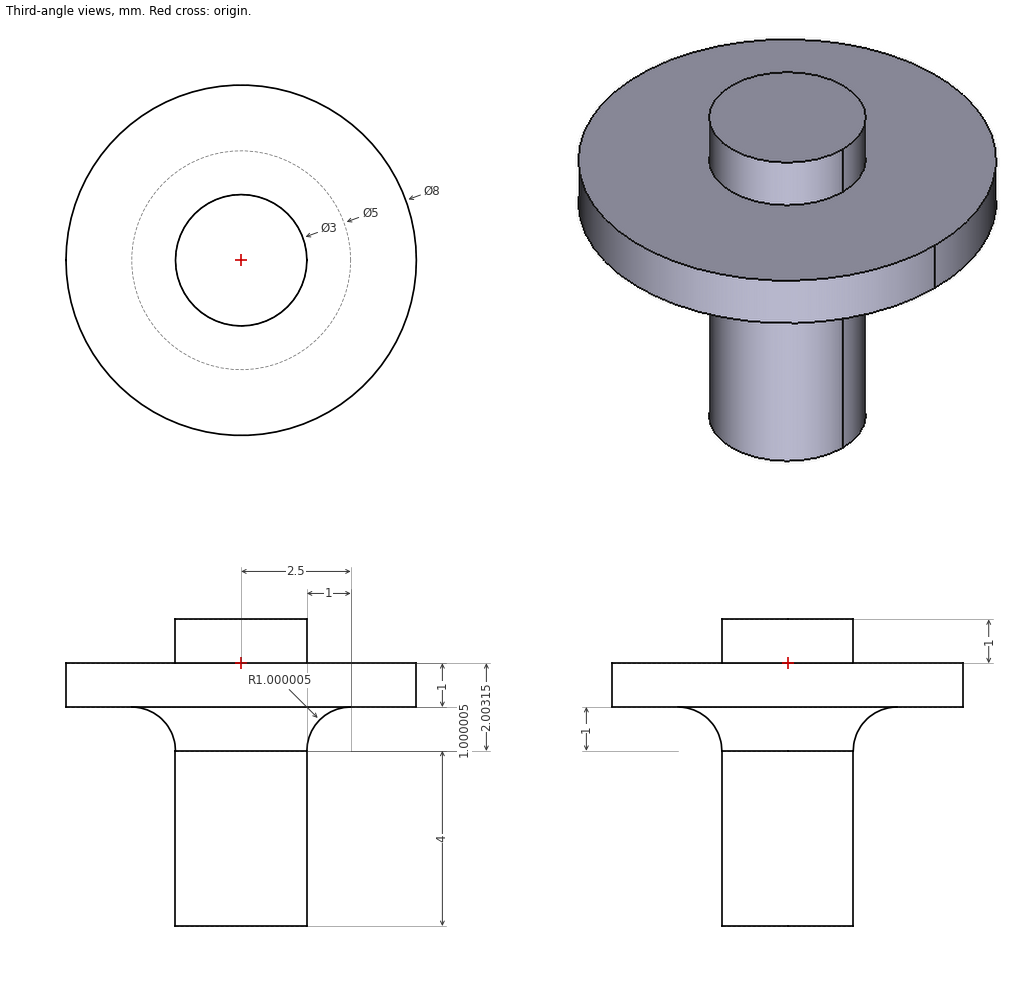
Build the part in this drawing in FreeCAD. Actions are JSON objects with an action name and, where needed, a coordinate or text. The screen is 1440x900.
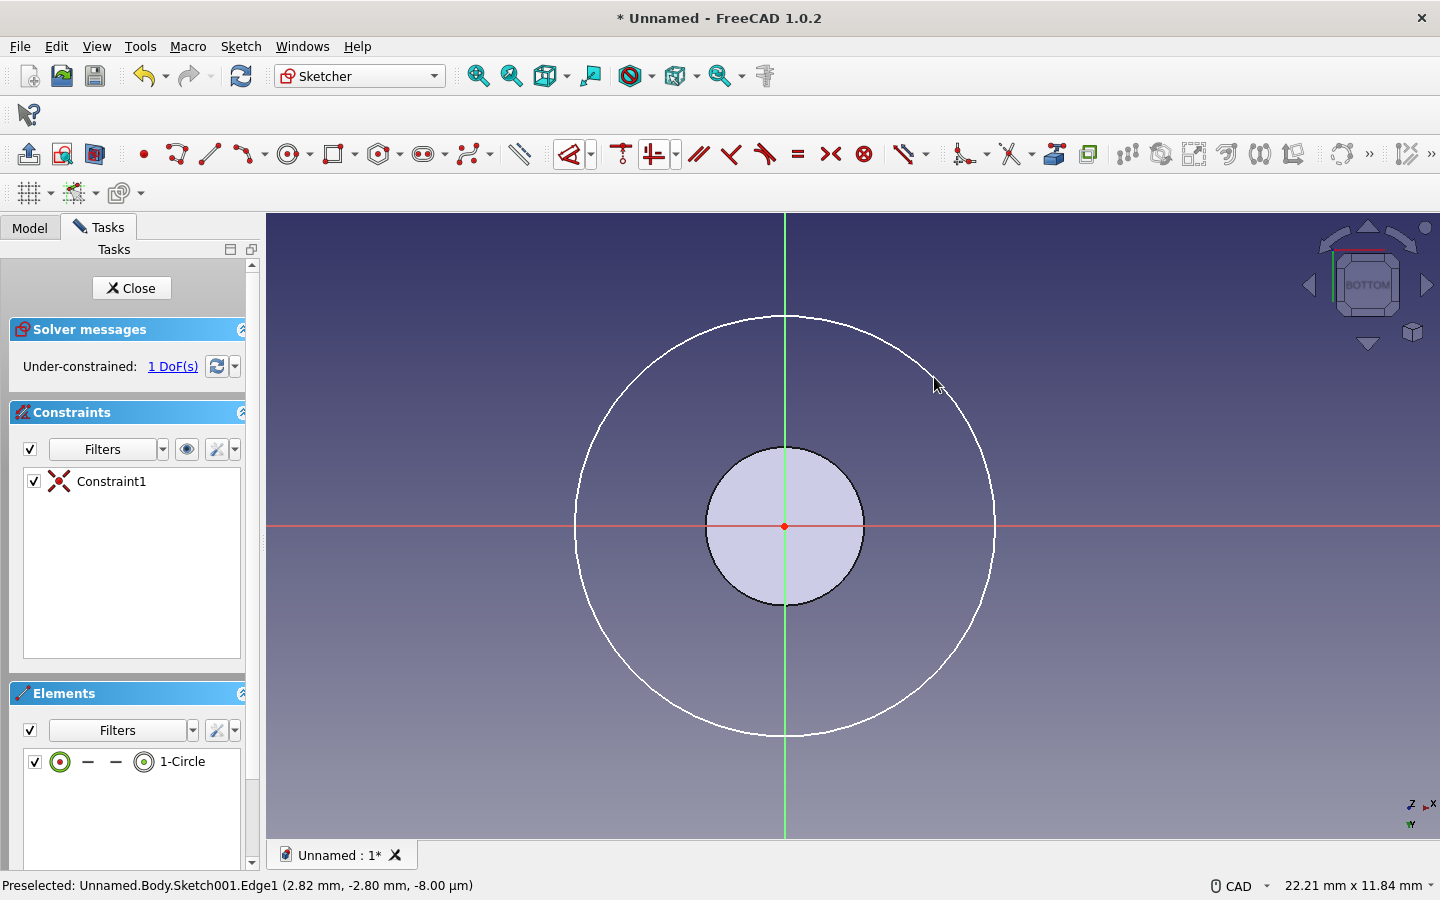
{"action": "left_click", "coordinate": [933, 377]}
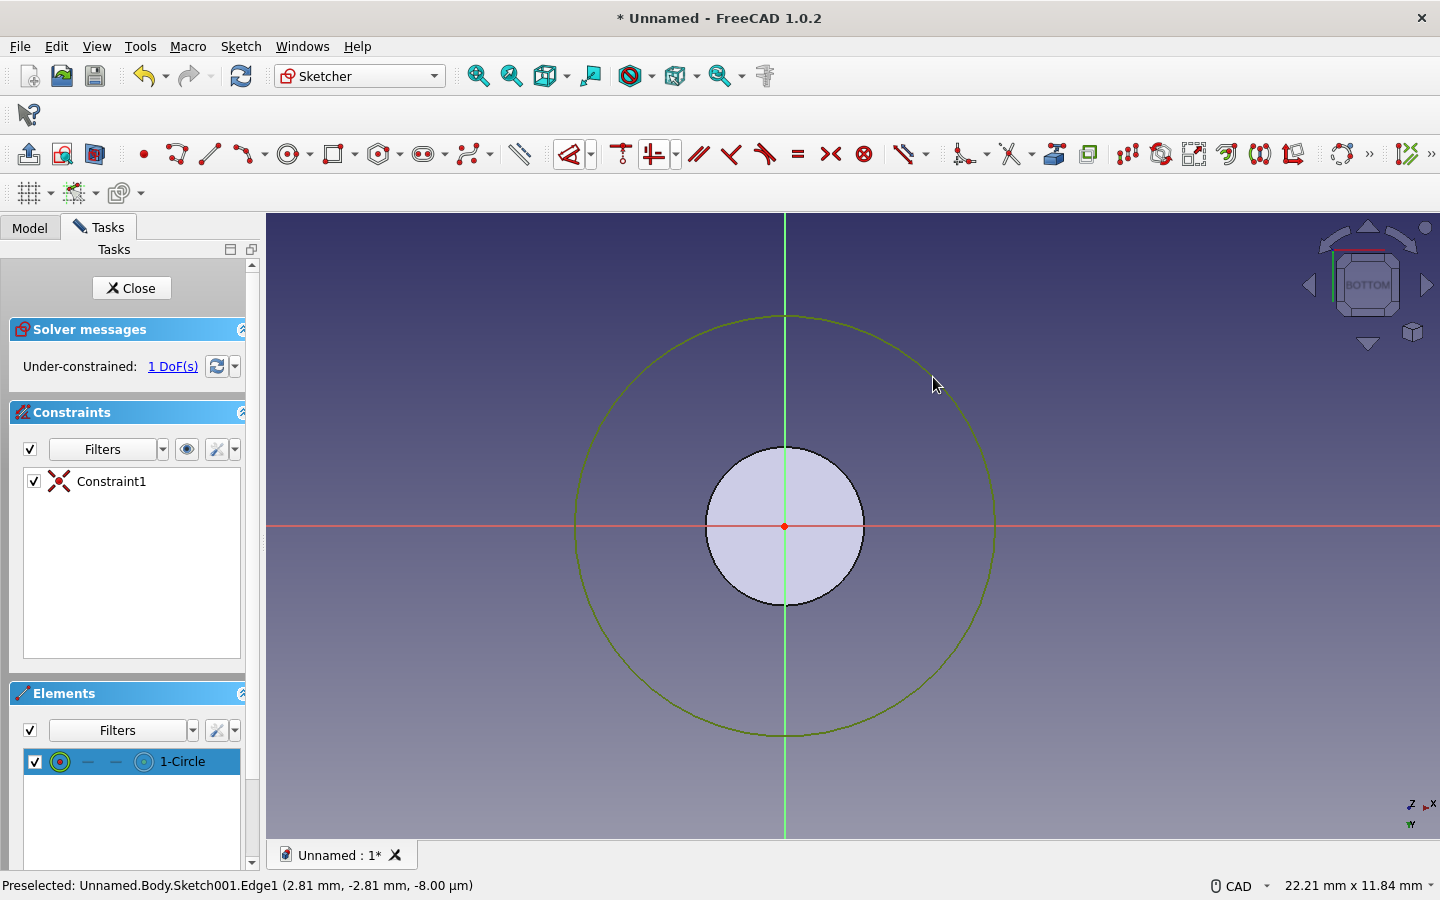
{"action": "key", "text": "k o"}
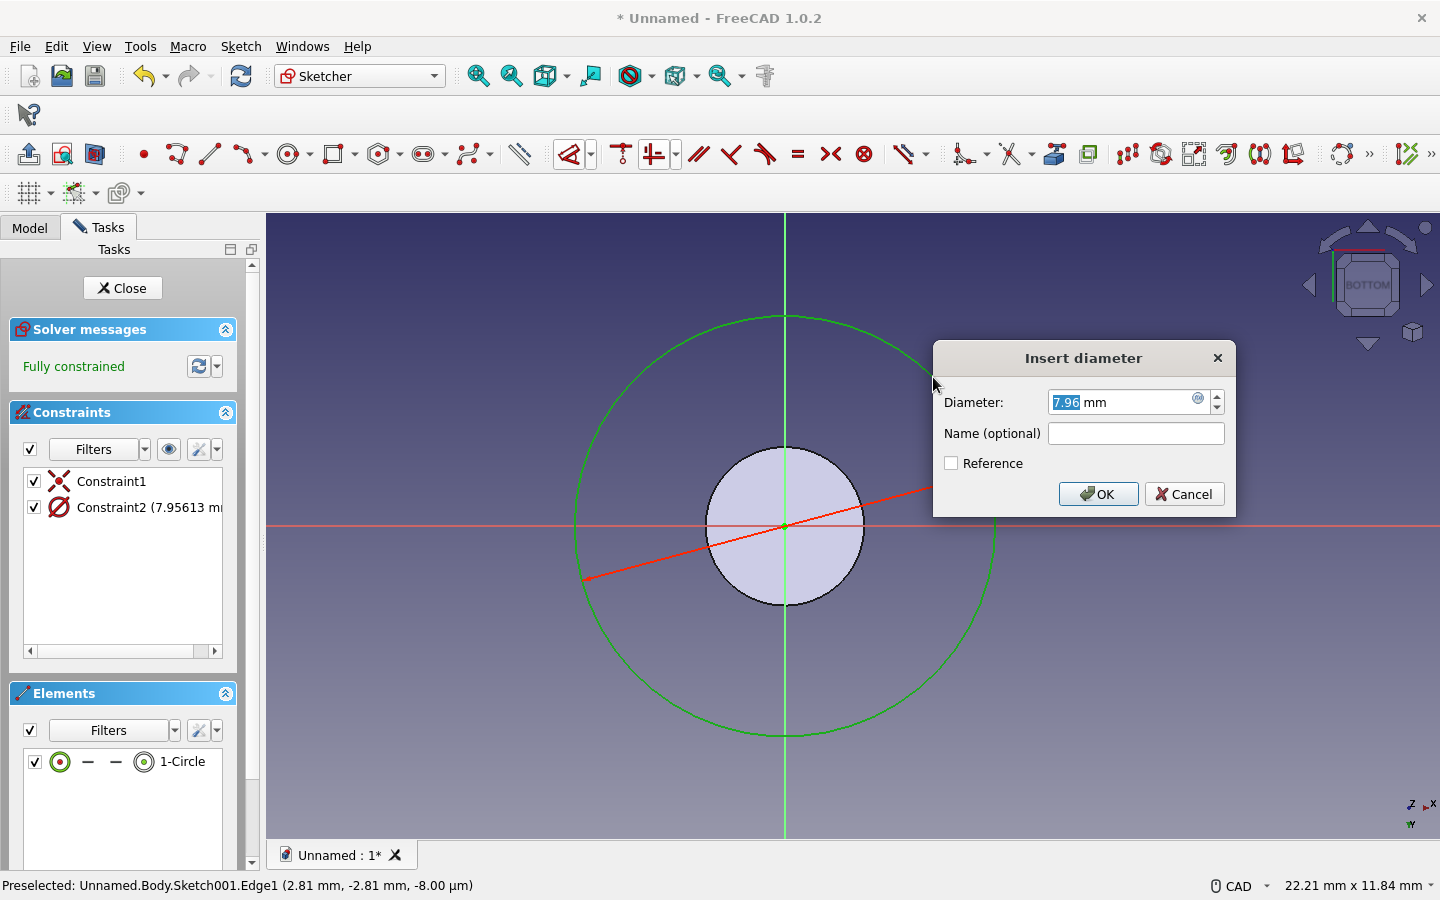
{"action": "type", "text": "8"}
{"action": "key", "text": "Return"}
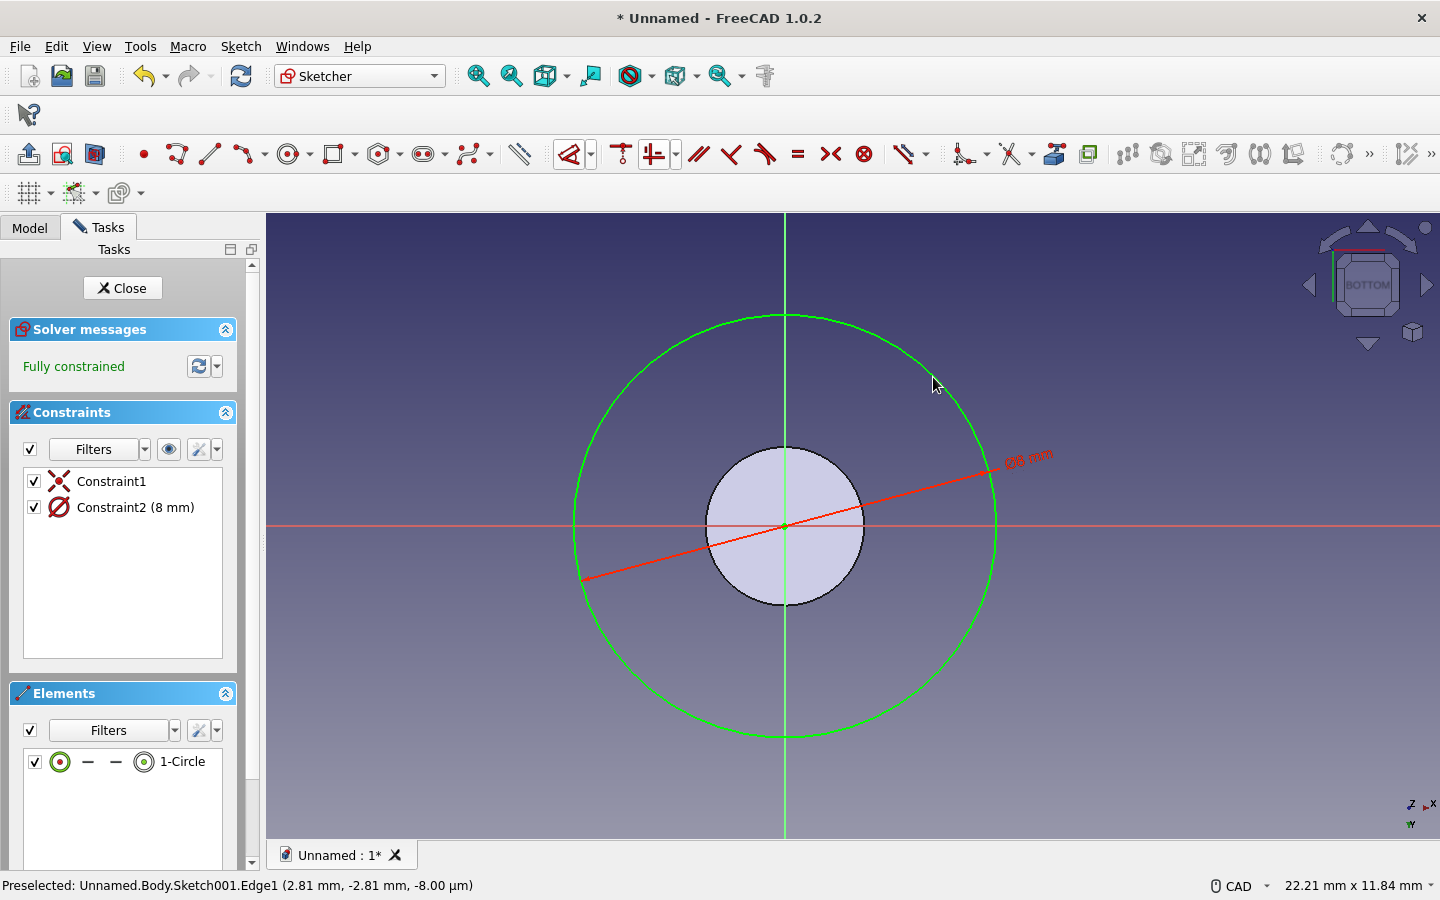
{"action": "left_click", "coordinate": [123, 288]}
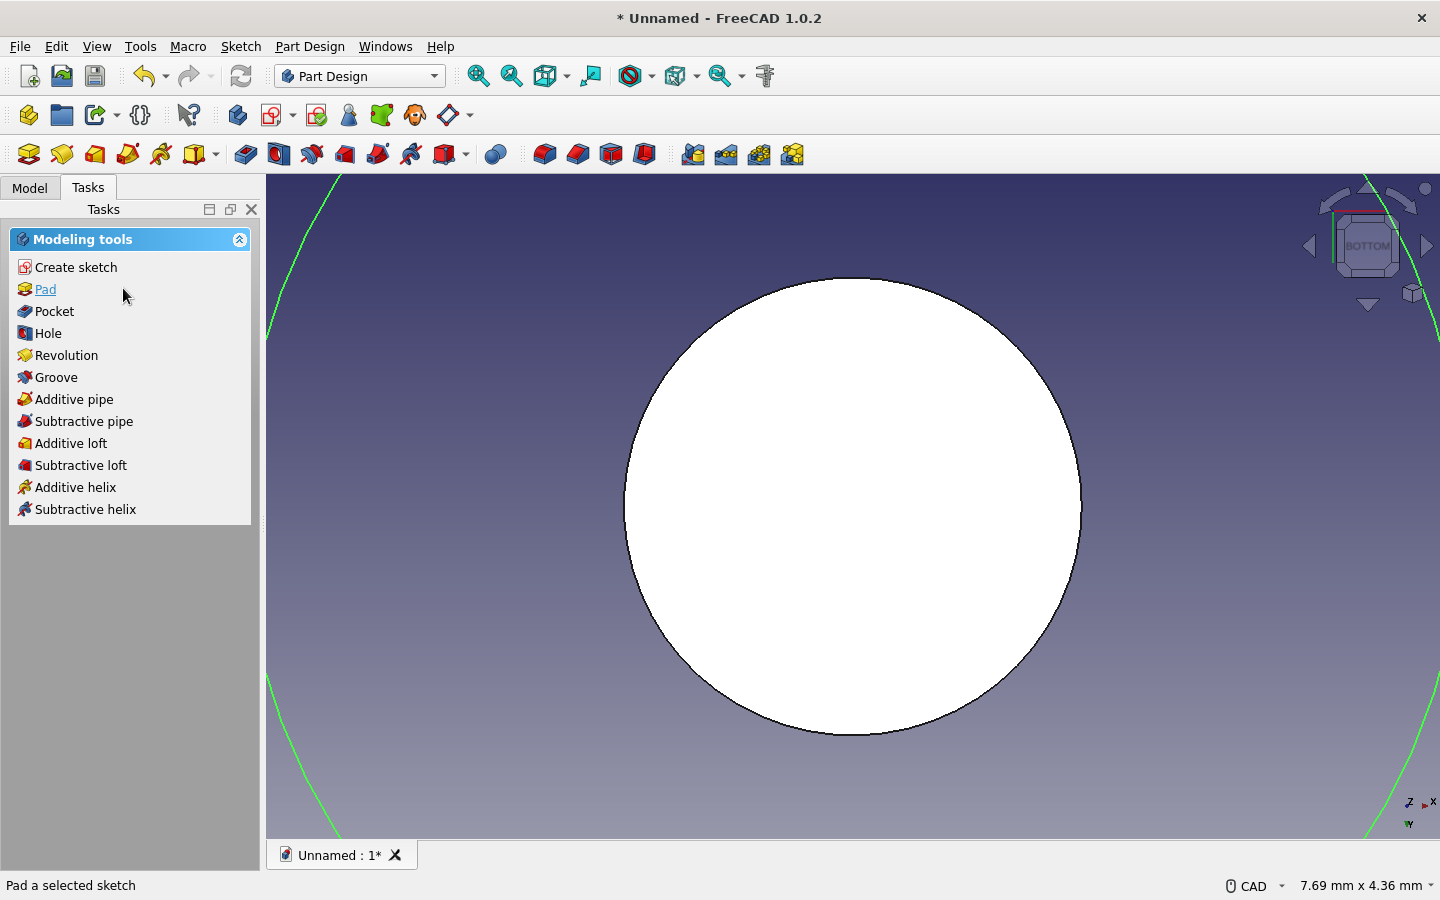
{"action": "left_click", "coordinate": [29, 154]}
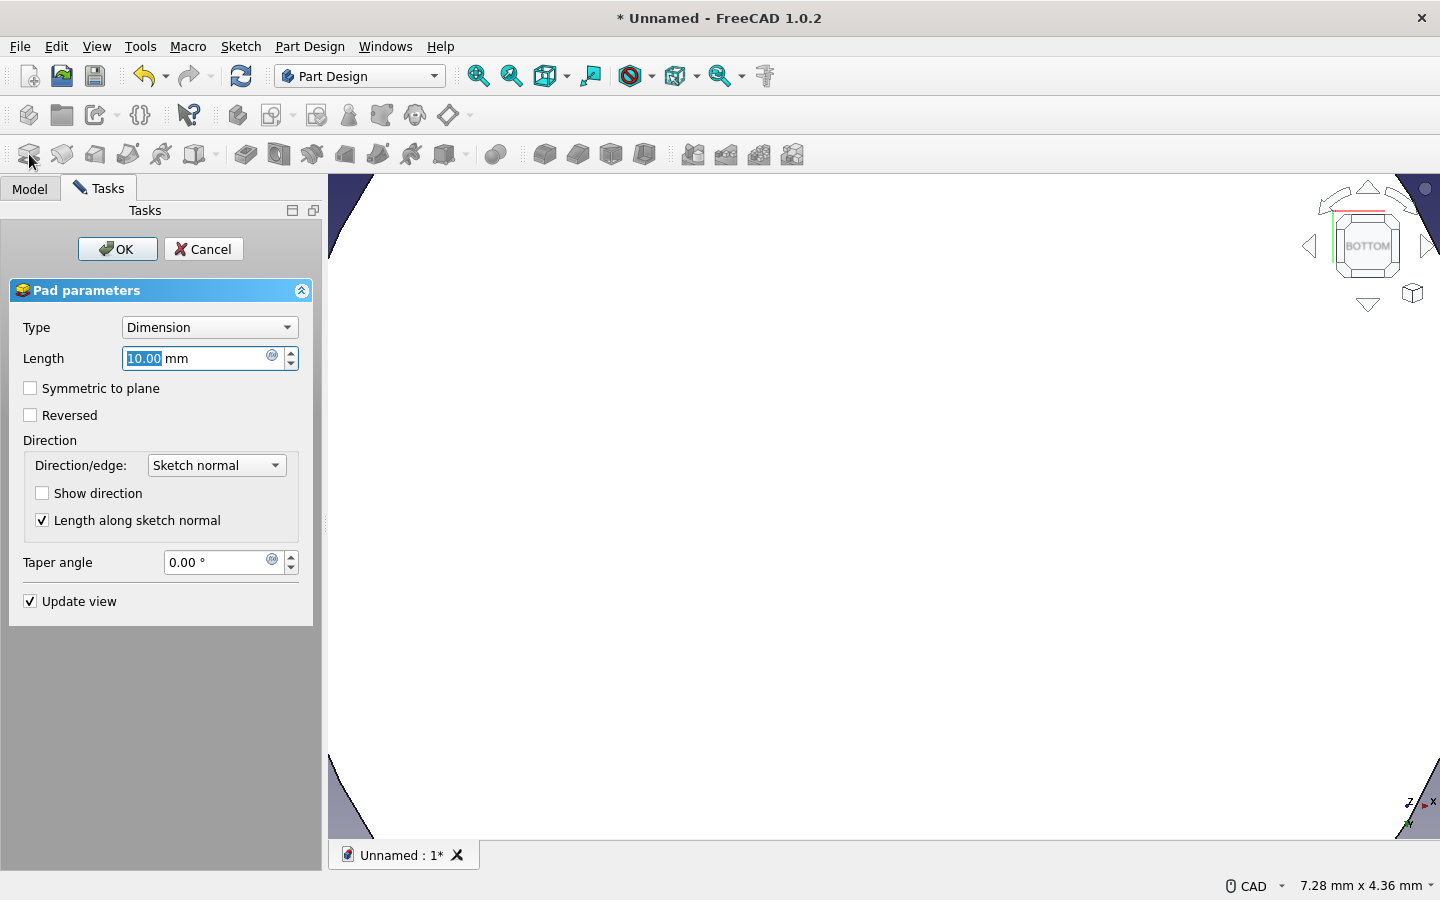
{"action": "type", "text": "1"}
{"action": "key", "text": "Tab"}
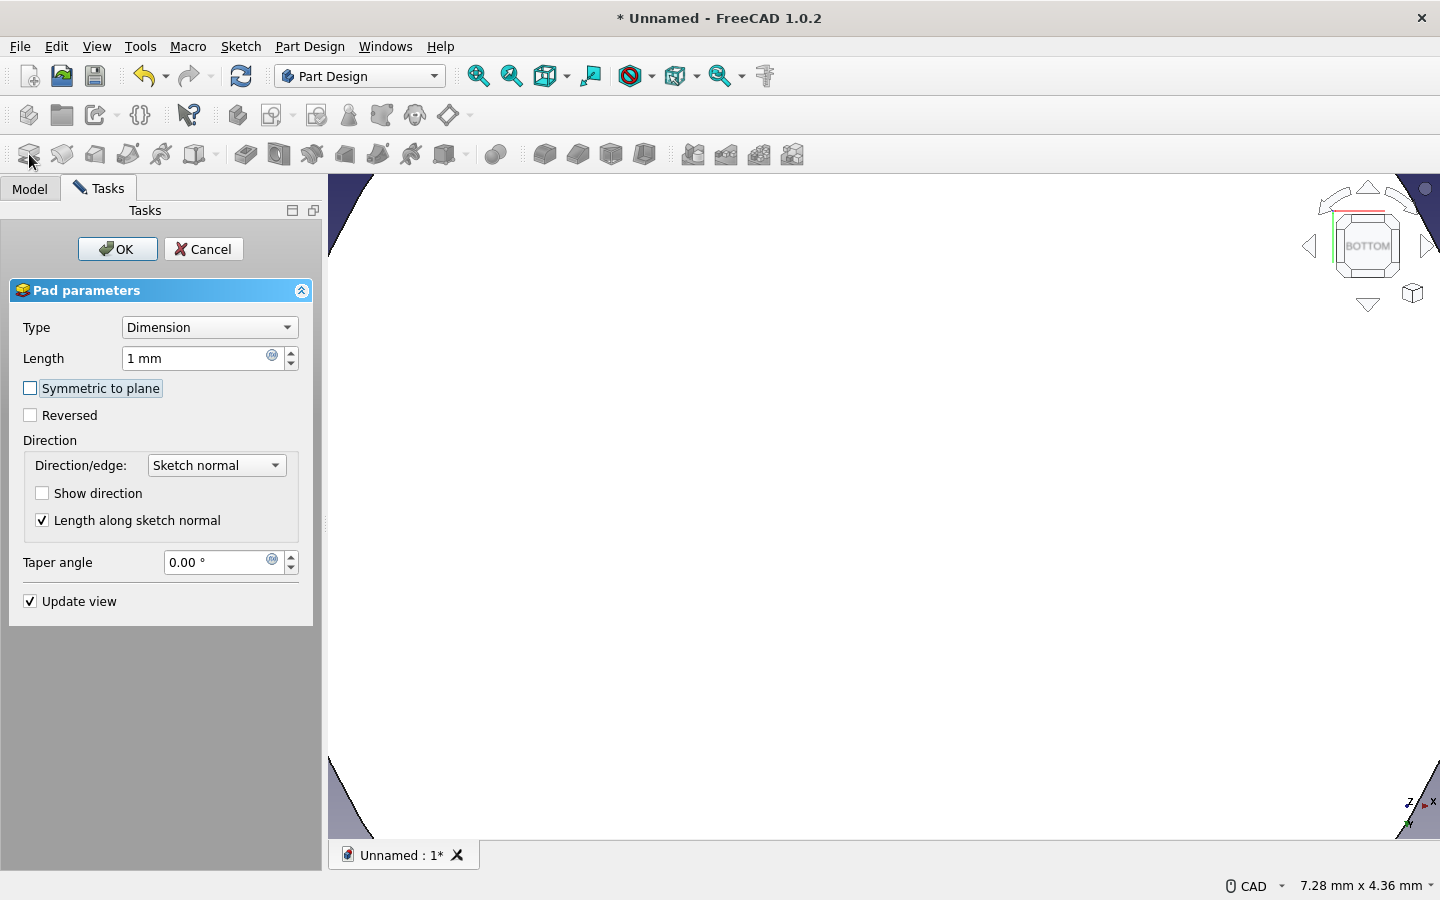
{"action": "left_click", "coordinate": [118, 249]}